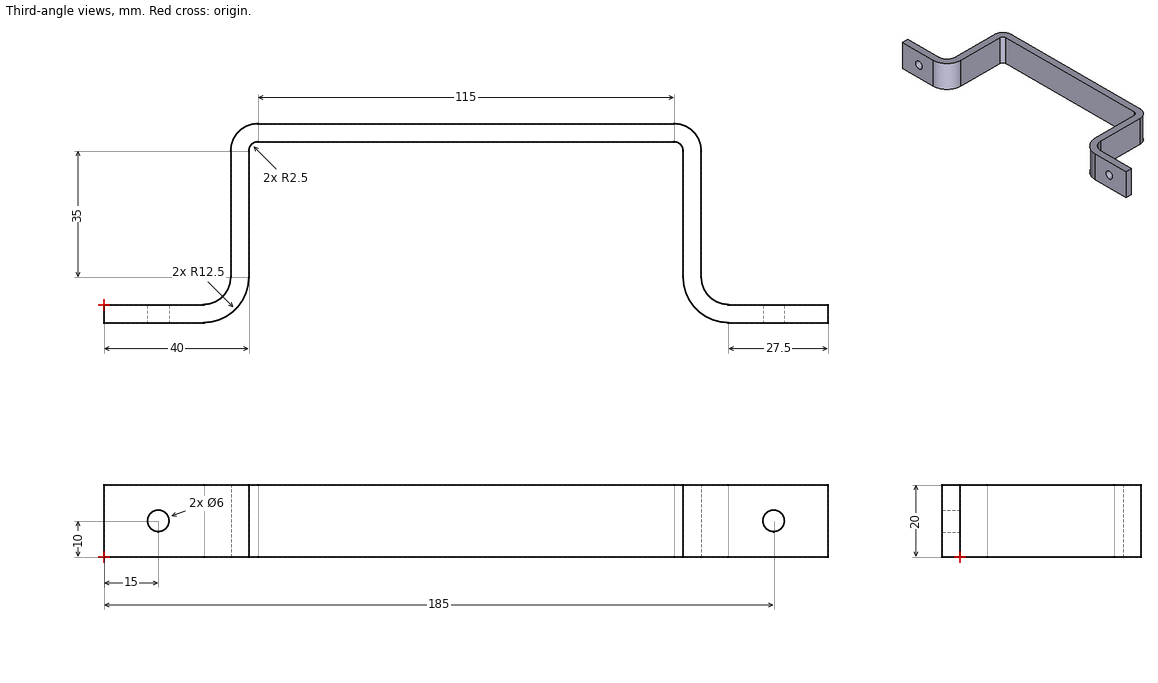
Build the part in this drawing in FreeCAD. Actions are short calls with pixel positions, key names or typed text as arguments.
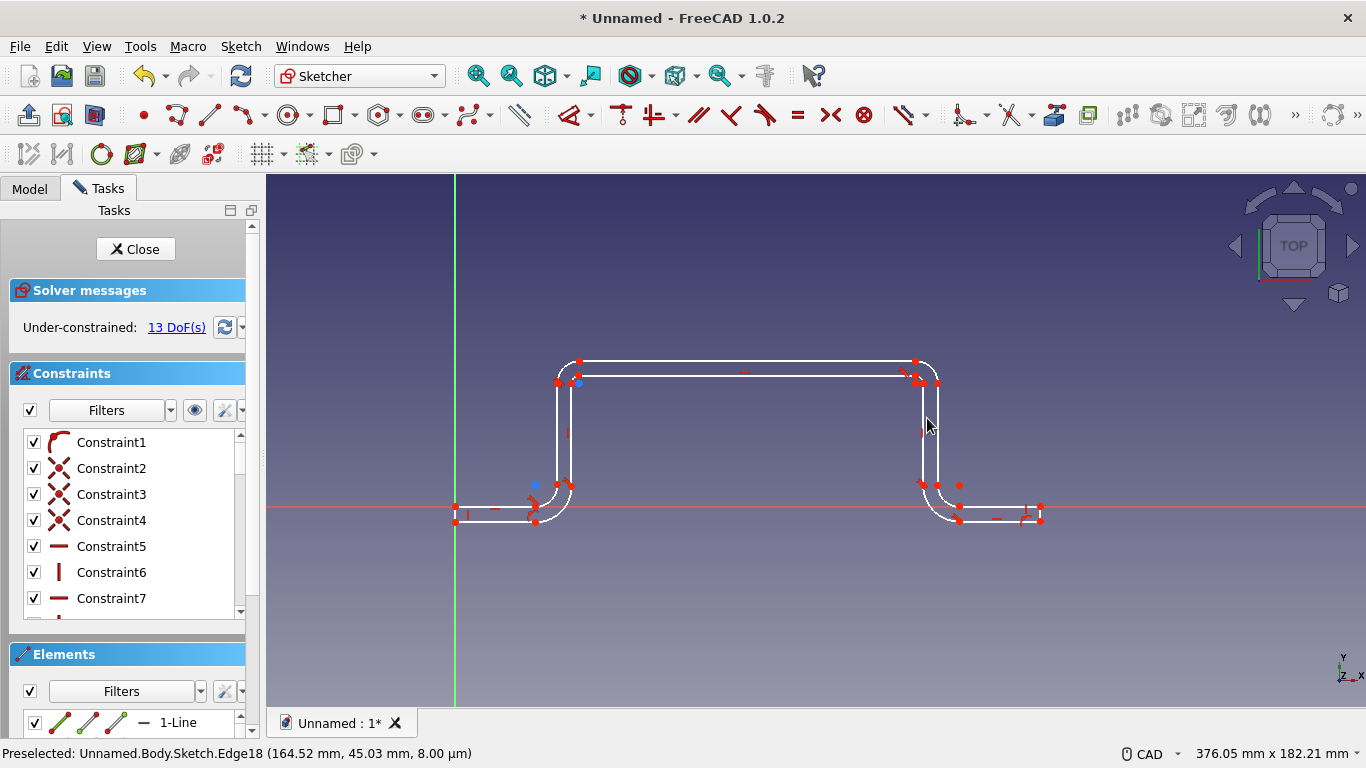
scroll(576, 377, up, 7)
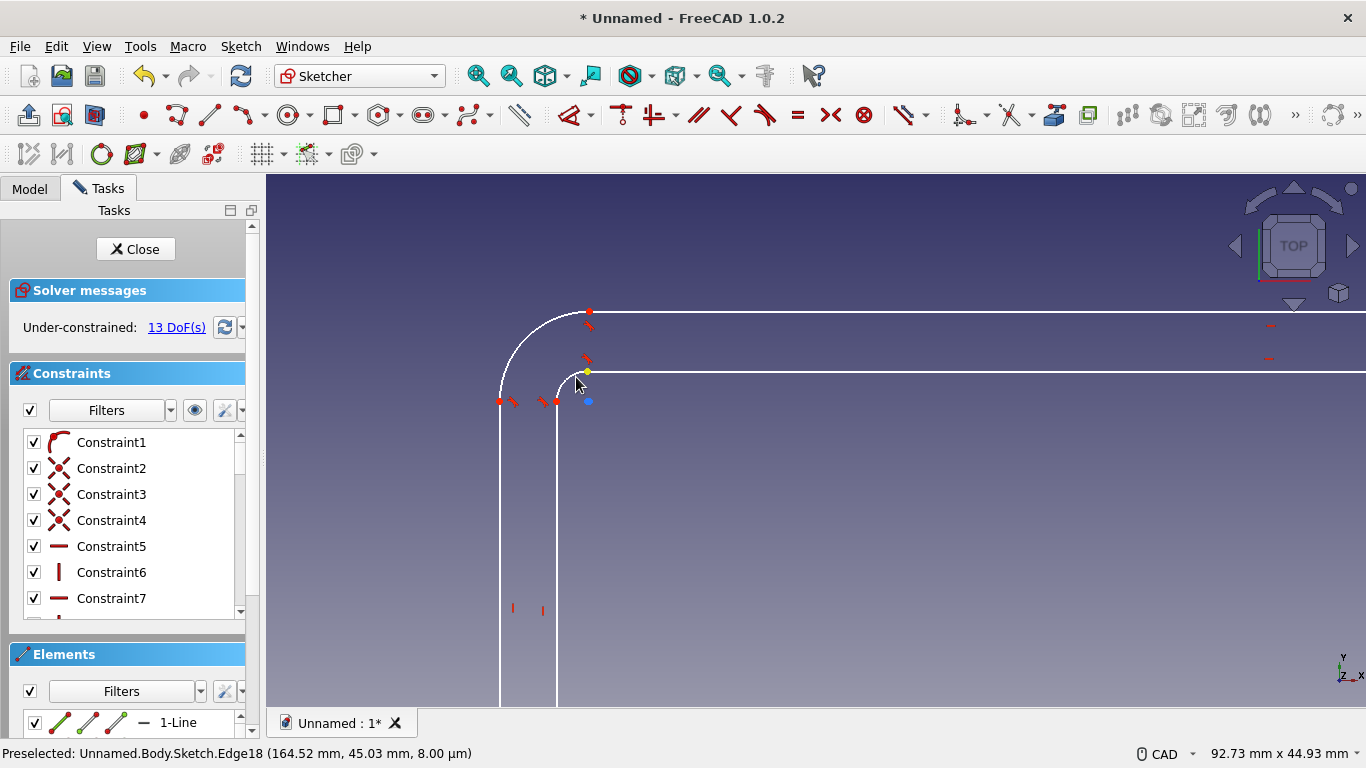
click(573, 375)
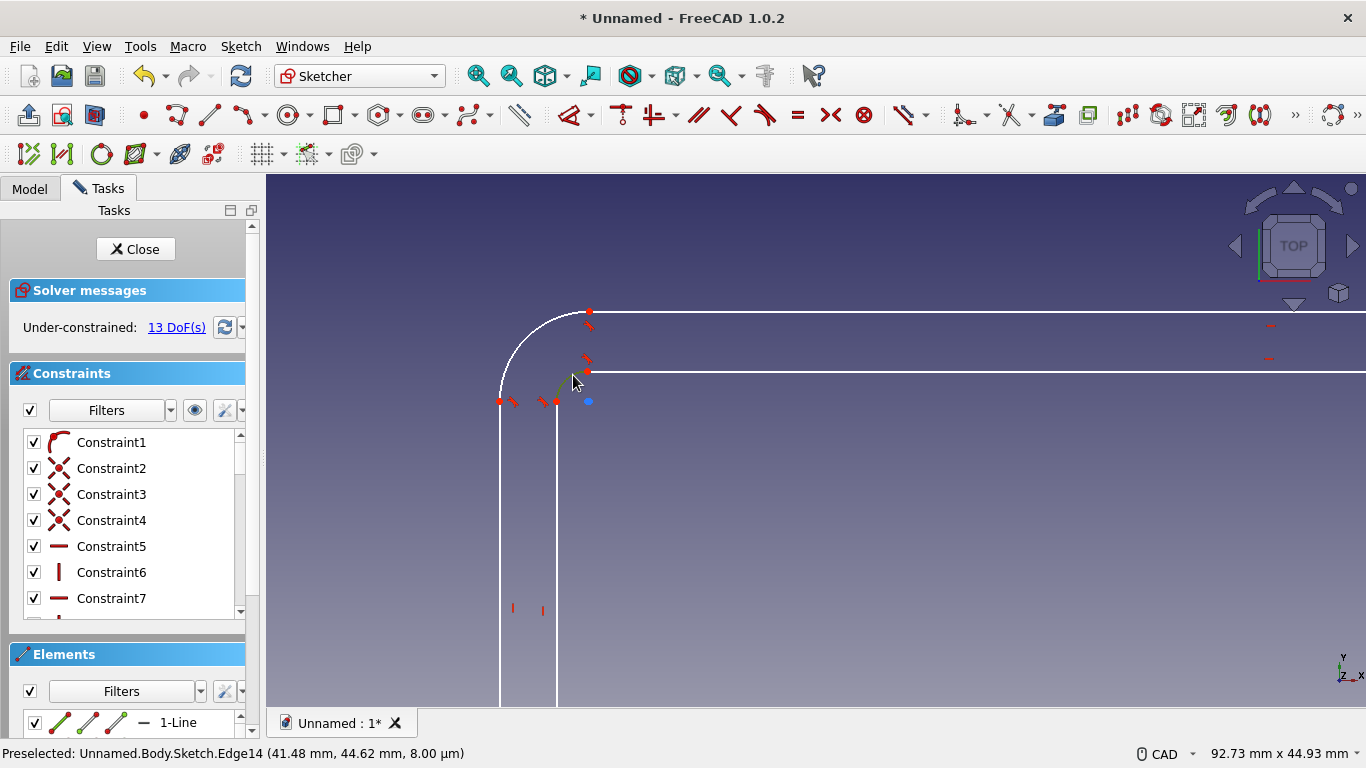
scroll(576, 377, down, 7)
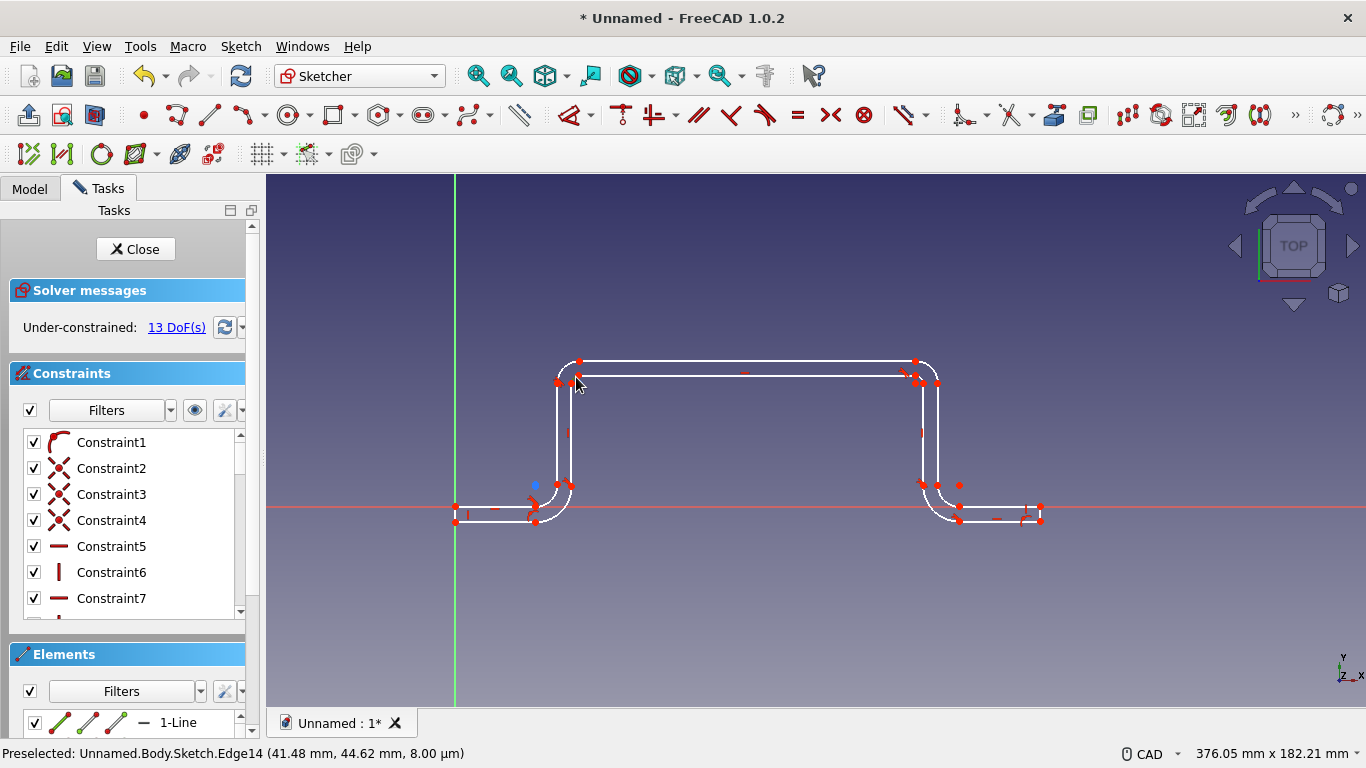
scroll(570, 364, up, 2)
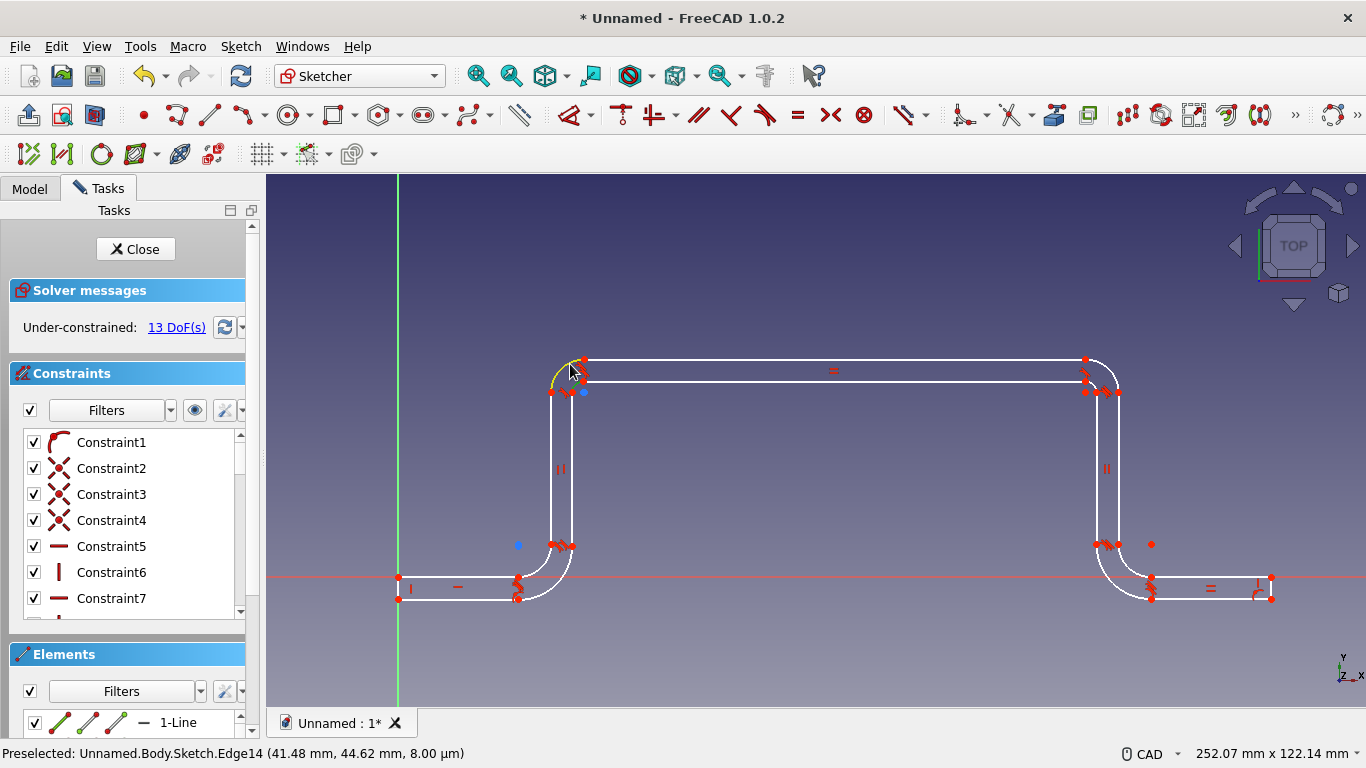
click(569, 363)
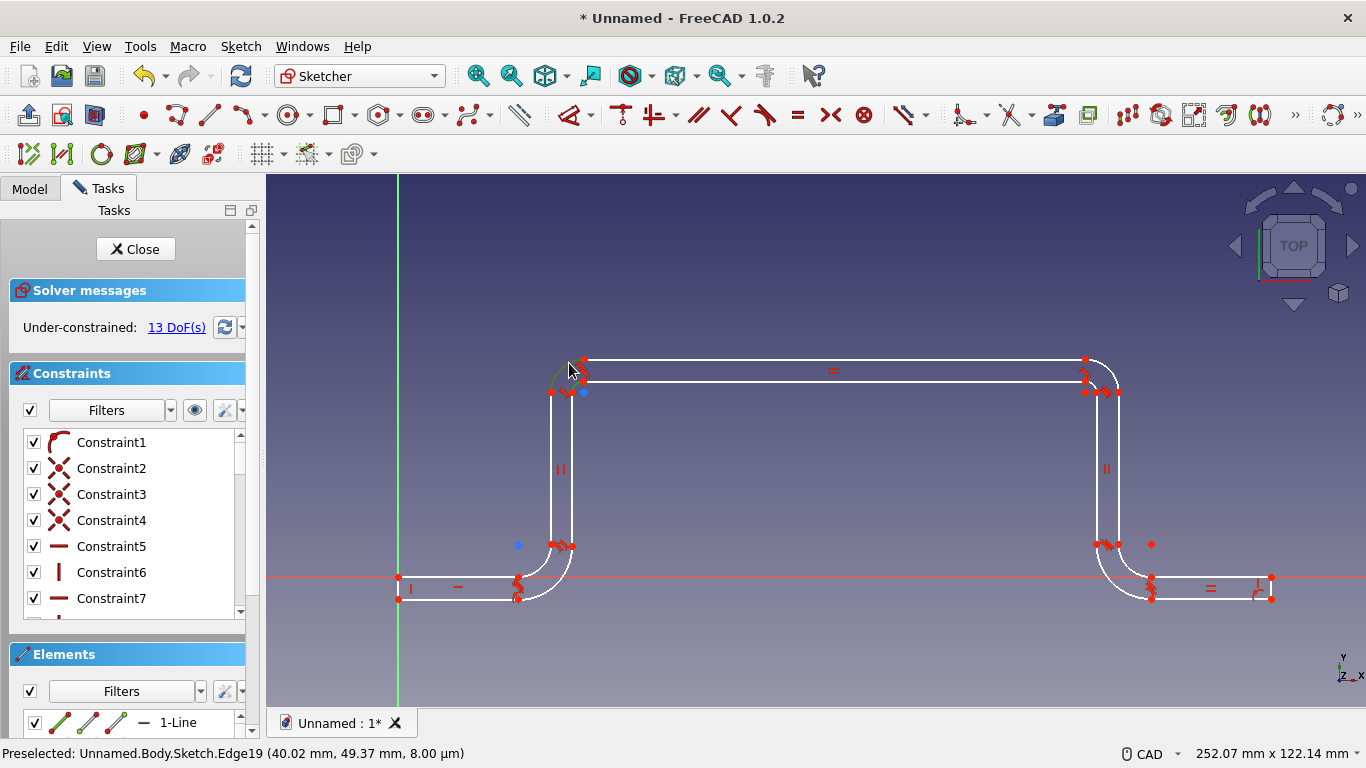
click(621, 116)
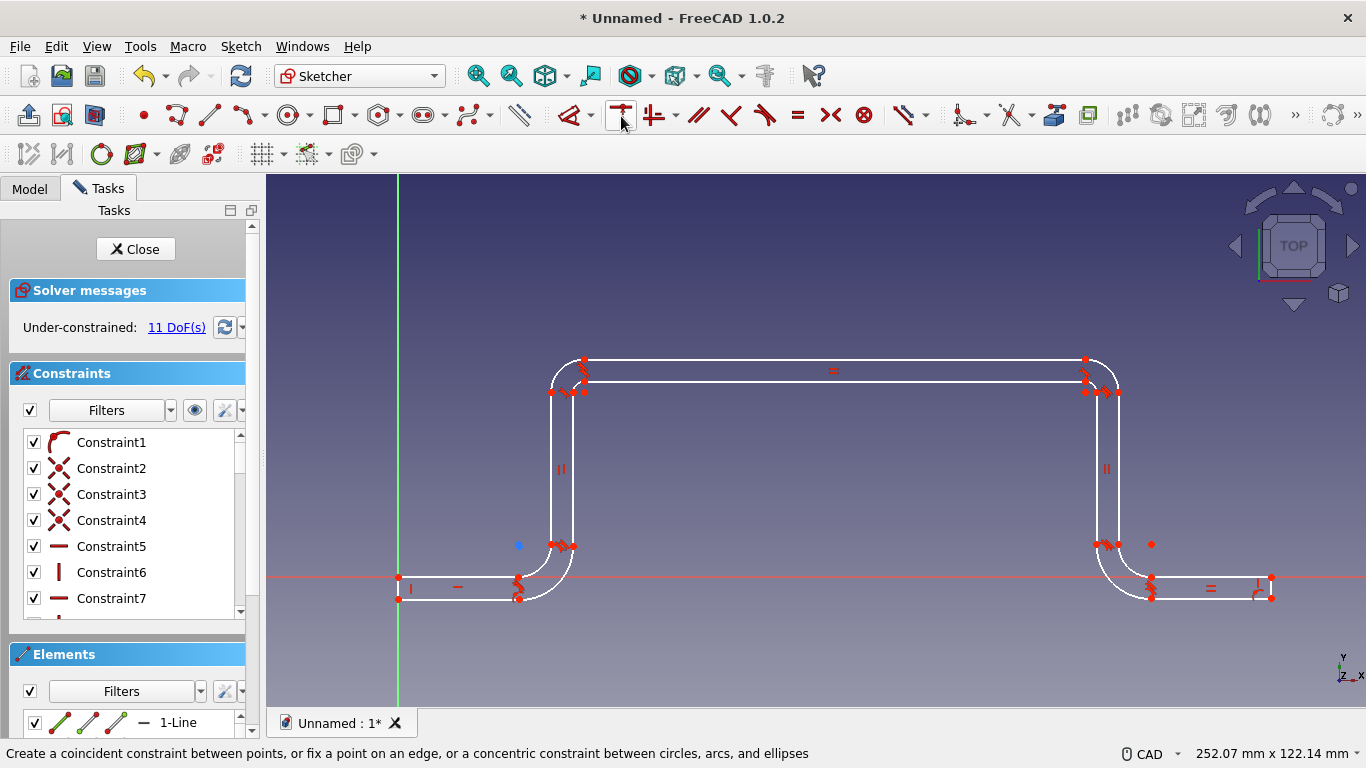
click(544, 594)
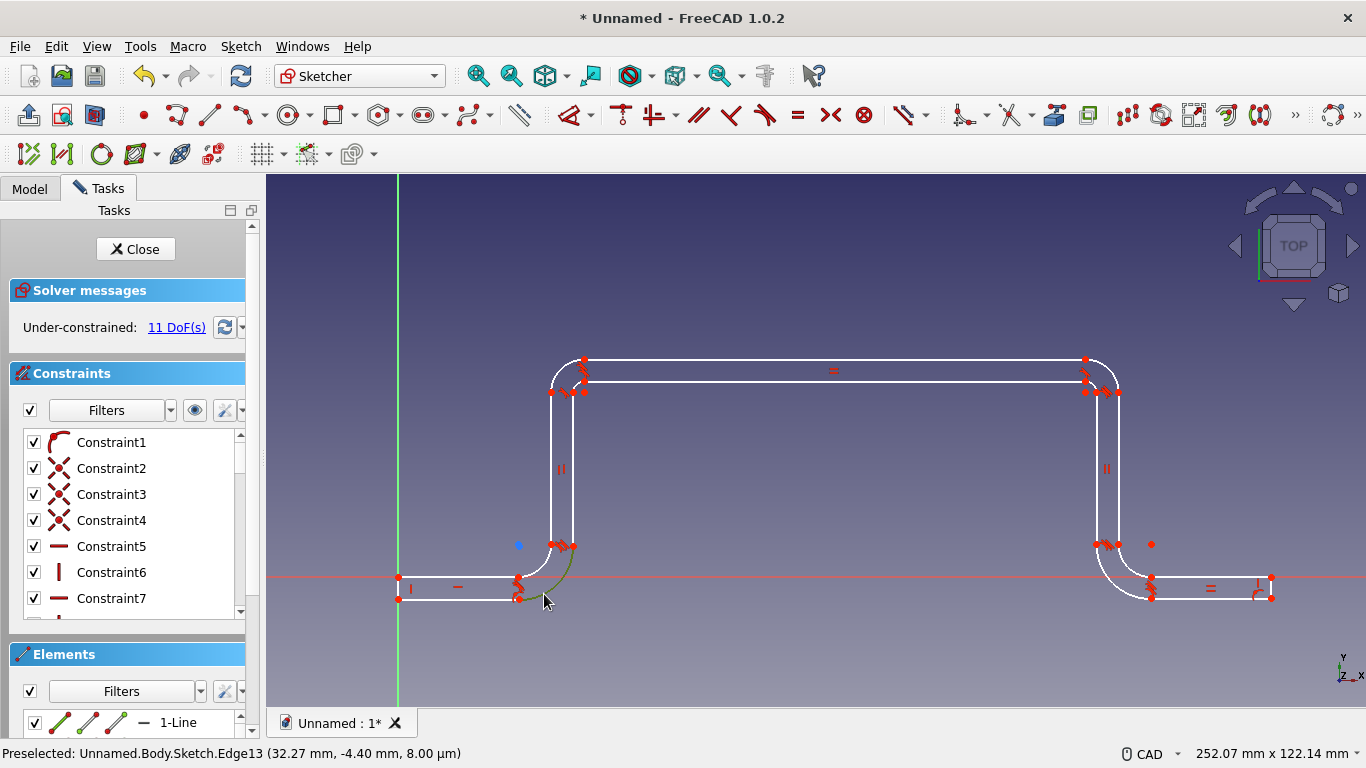
click(533, 573)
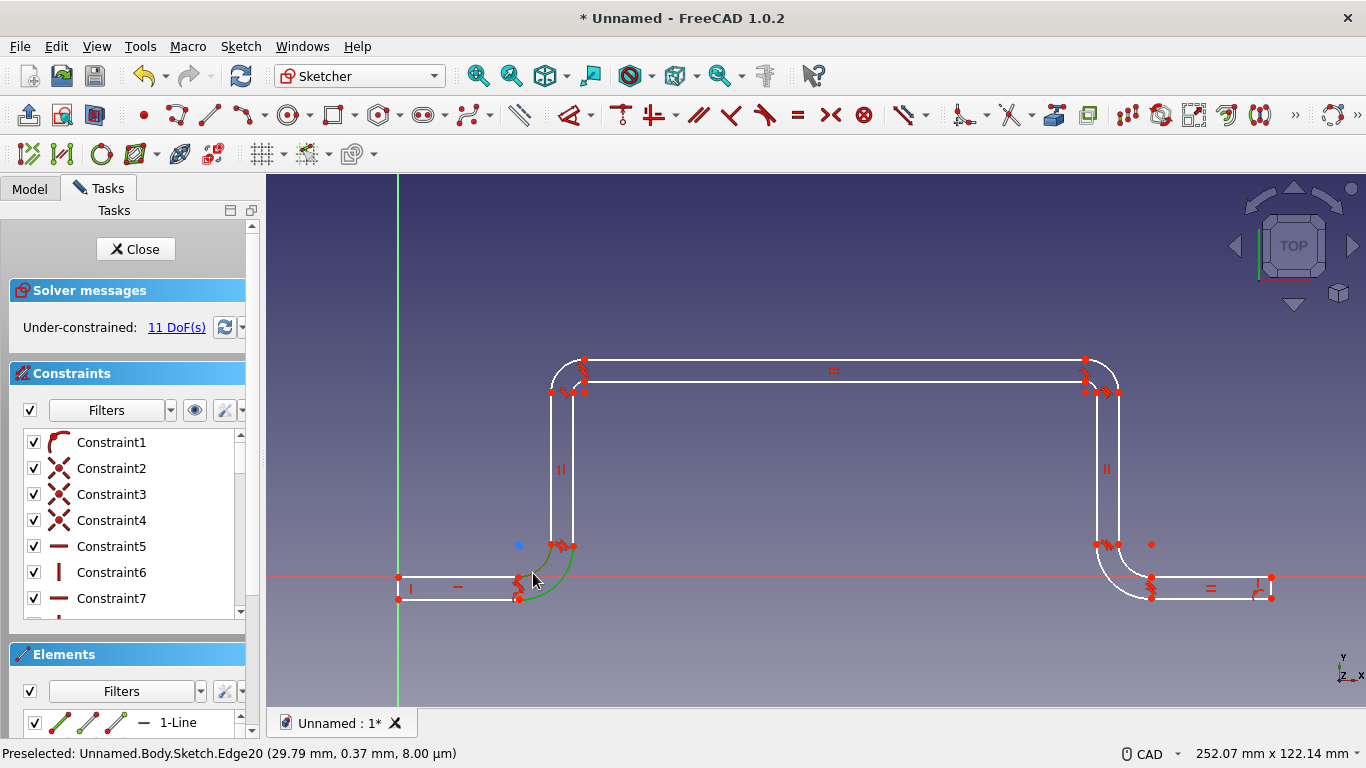
key(c)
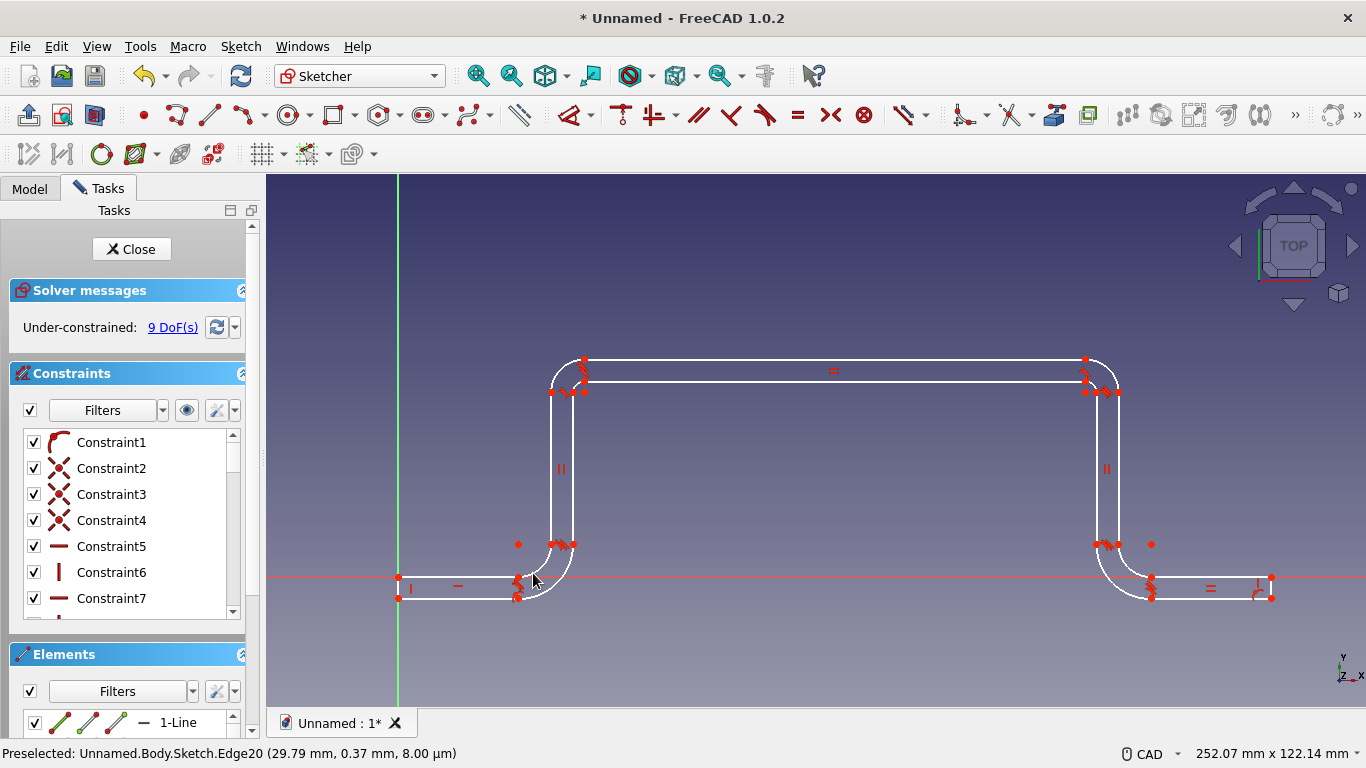
scroll(576, 385, up, 3)